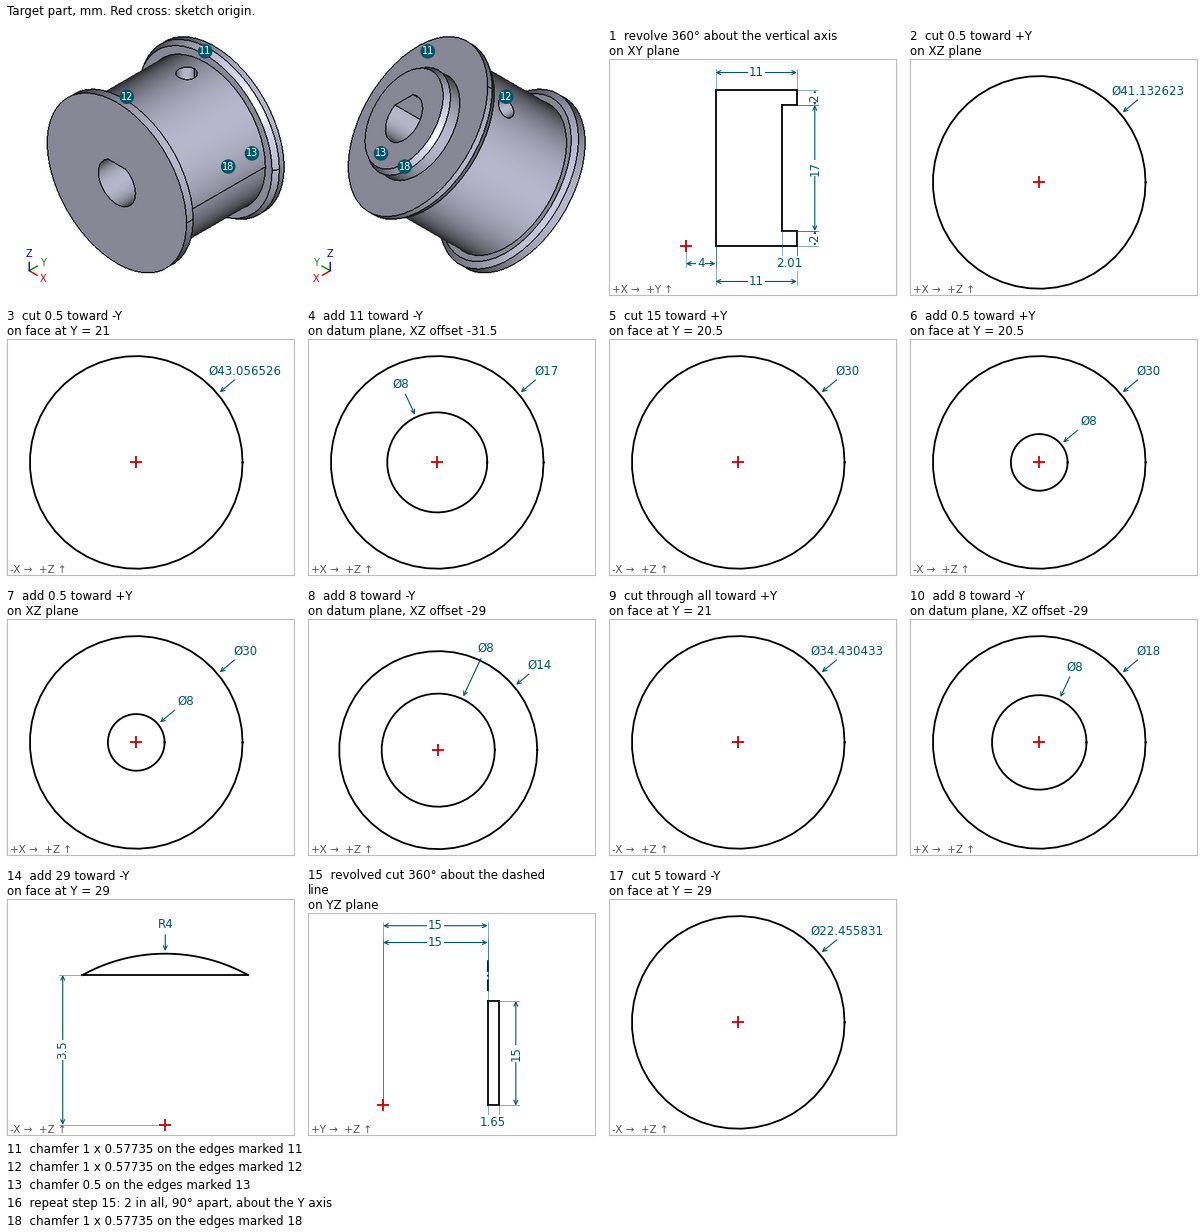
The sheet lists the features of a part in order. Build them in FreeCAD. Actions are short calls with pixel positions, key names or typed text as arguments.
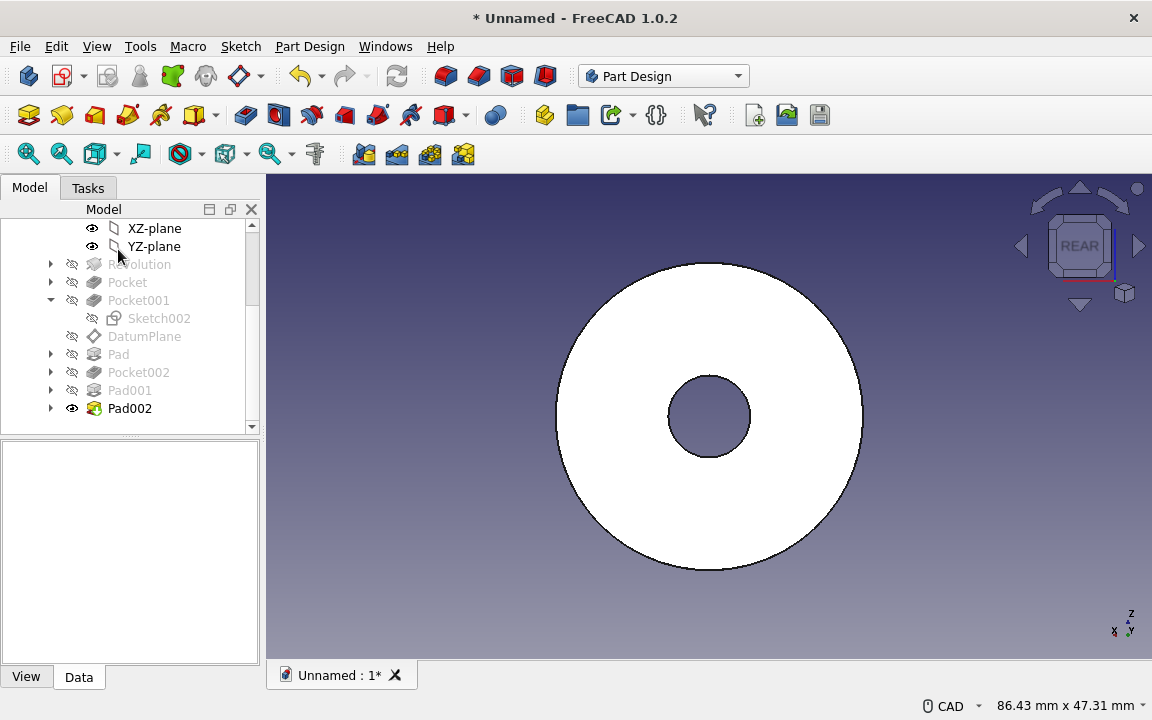
scroll(161, 314, down, 3)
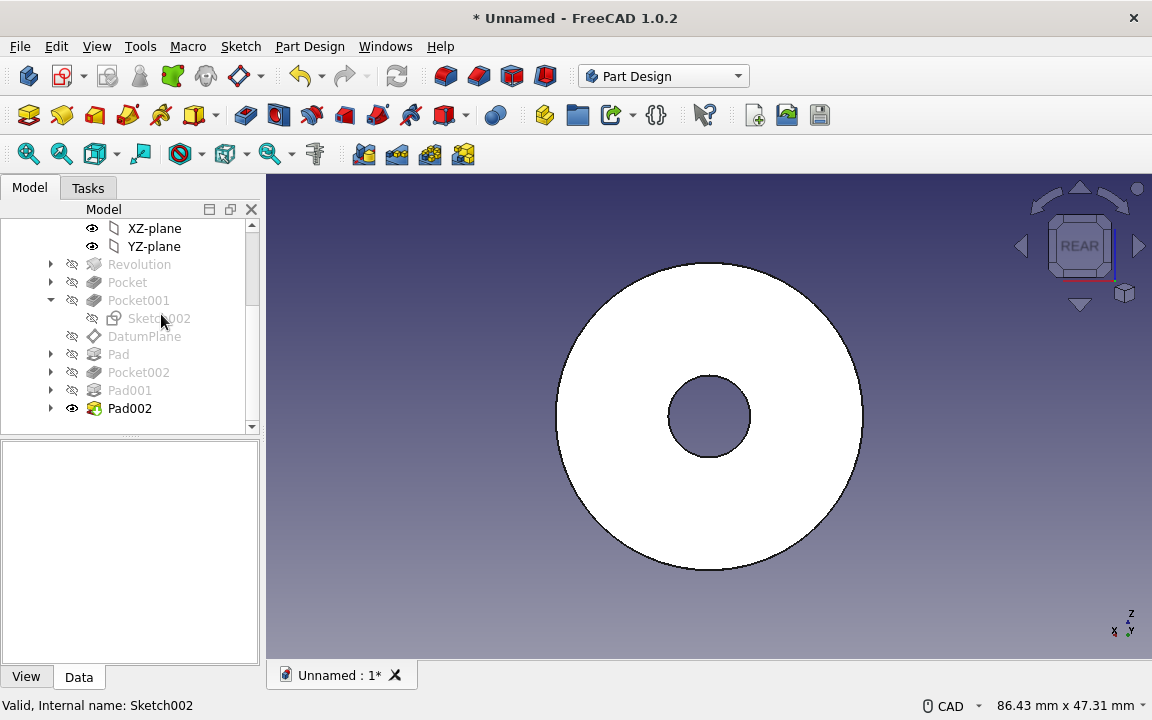
scroll(161, 314, up, 15)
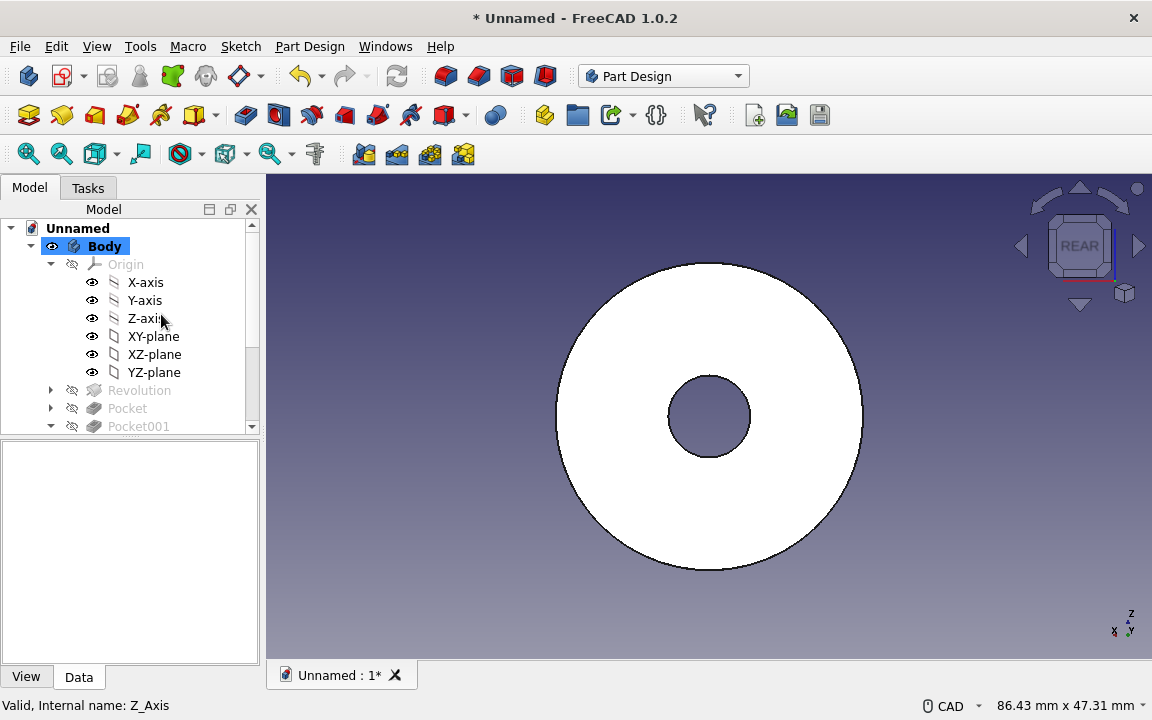
click(137, 354)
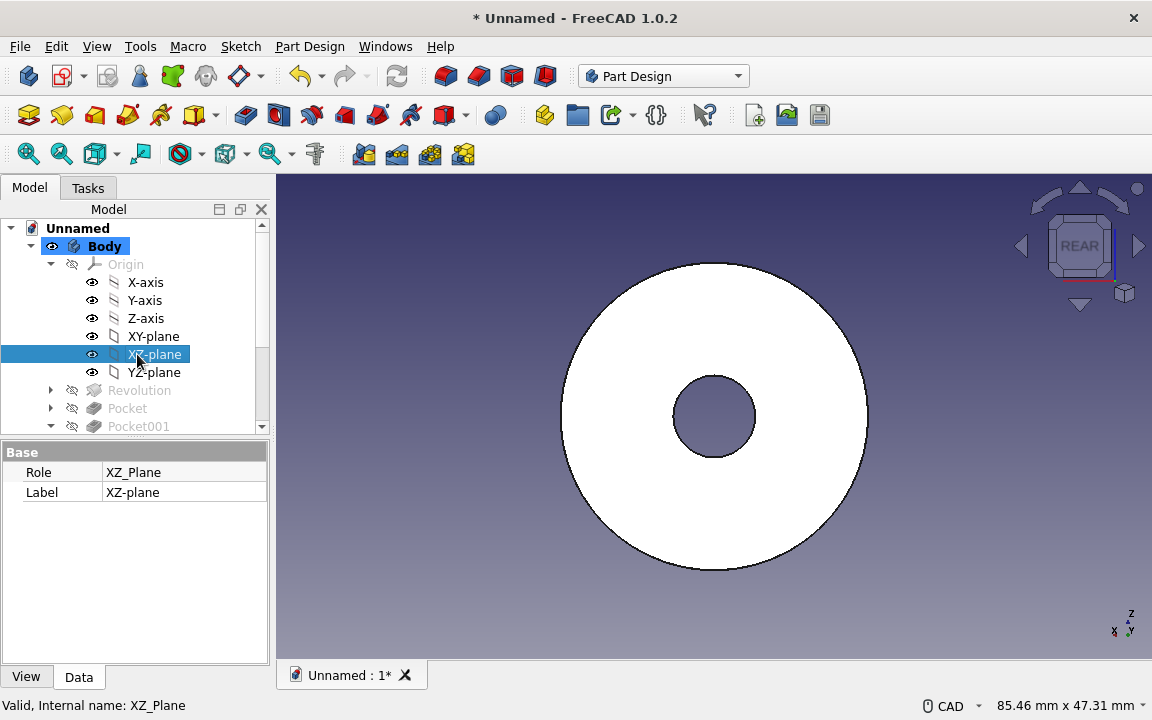
click(238, 76)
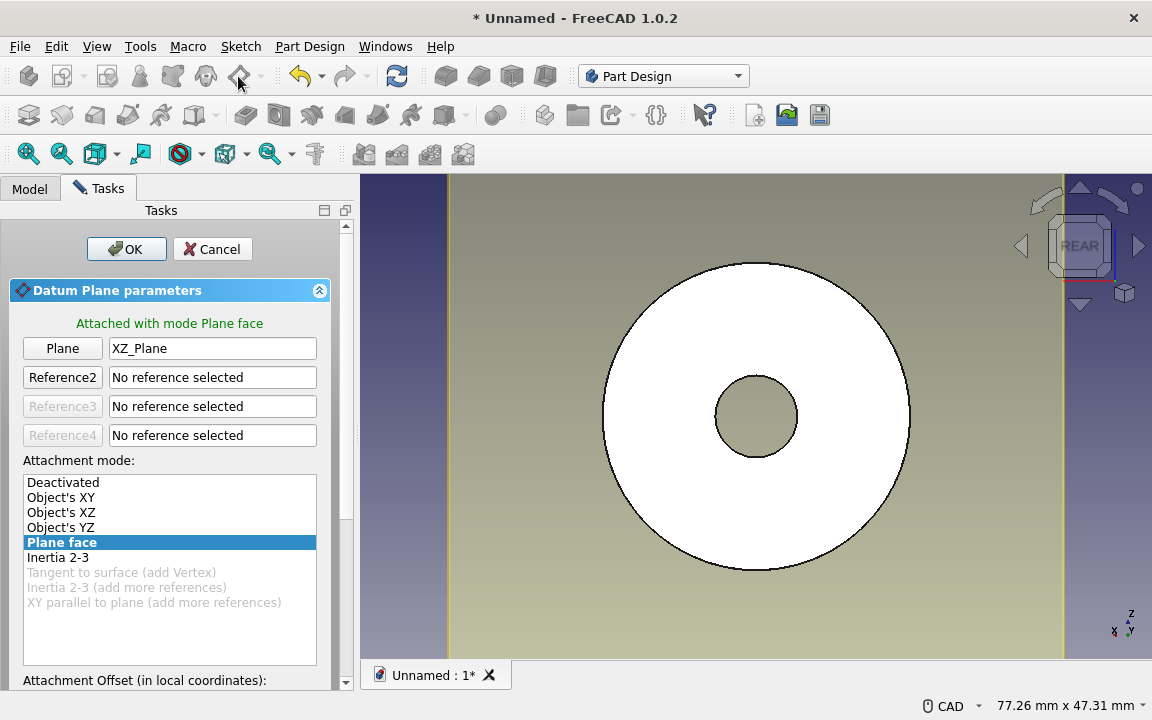
scroll(346, 455, down, 3)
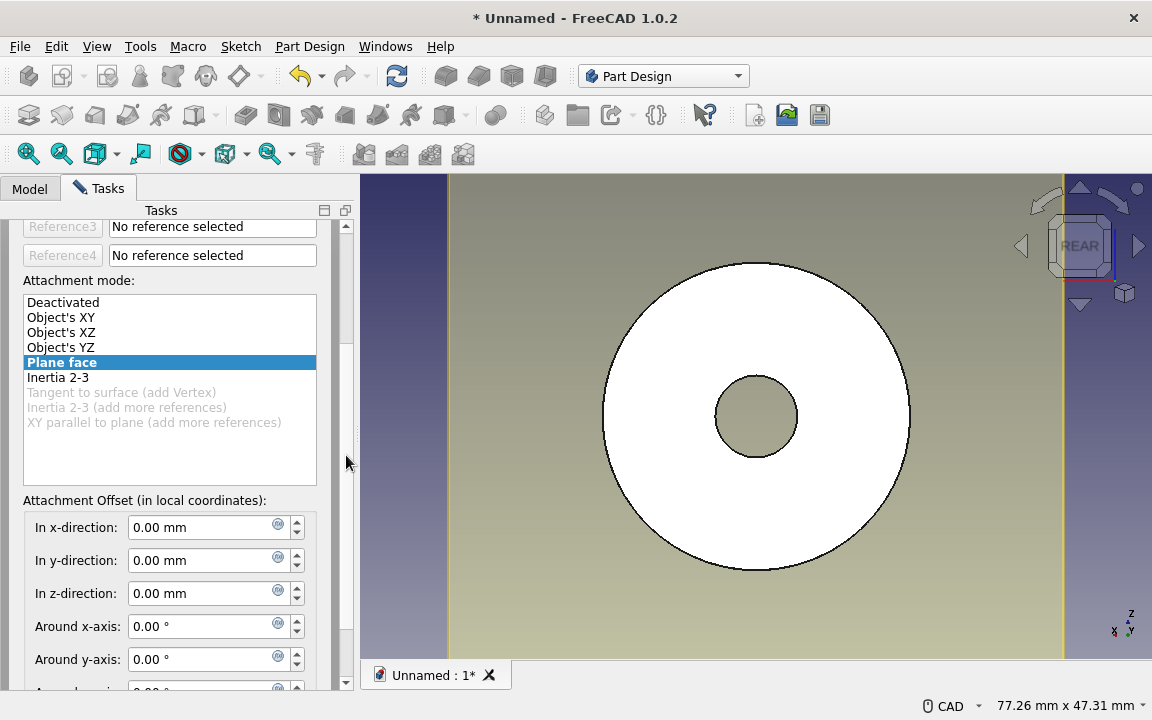
triple_click(210, 594)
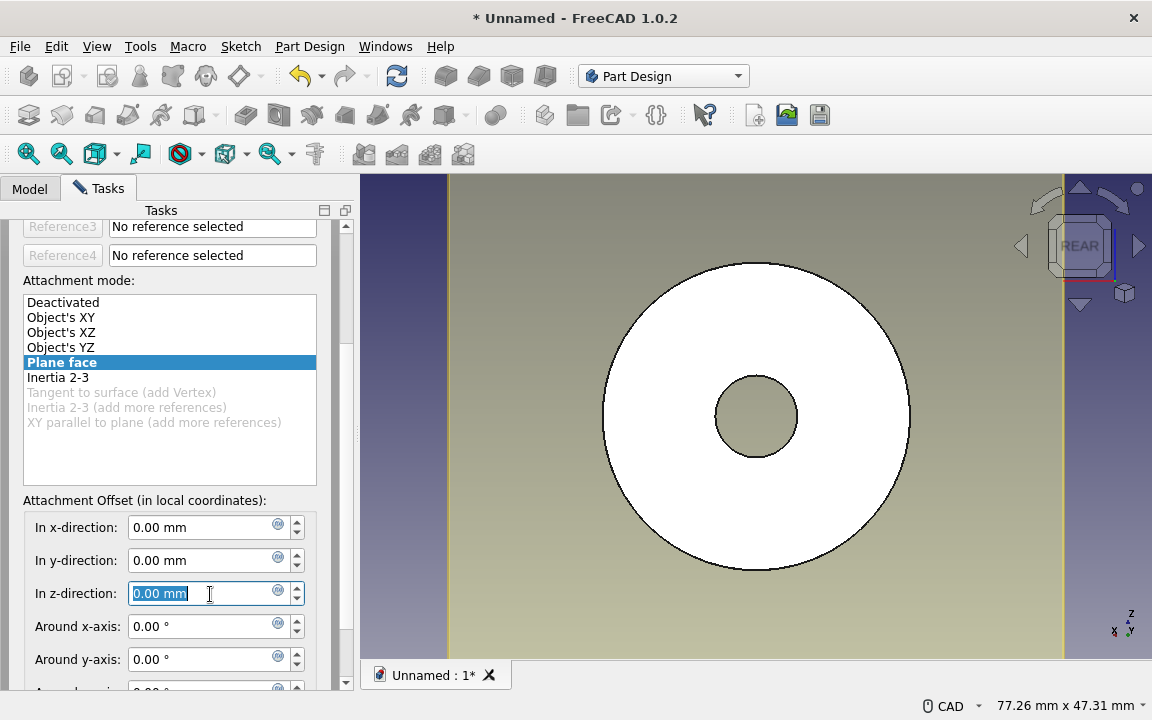
text(-29)
key(Tab)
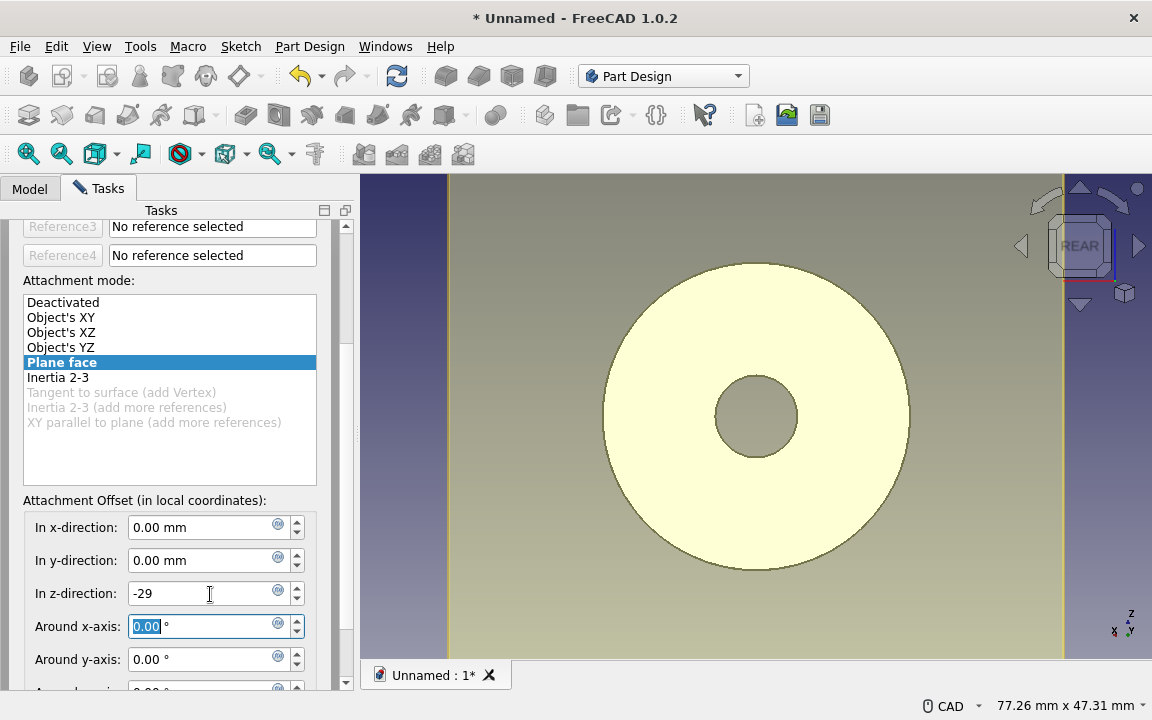
scroll(346, 455, up, 4)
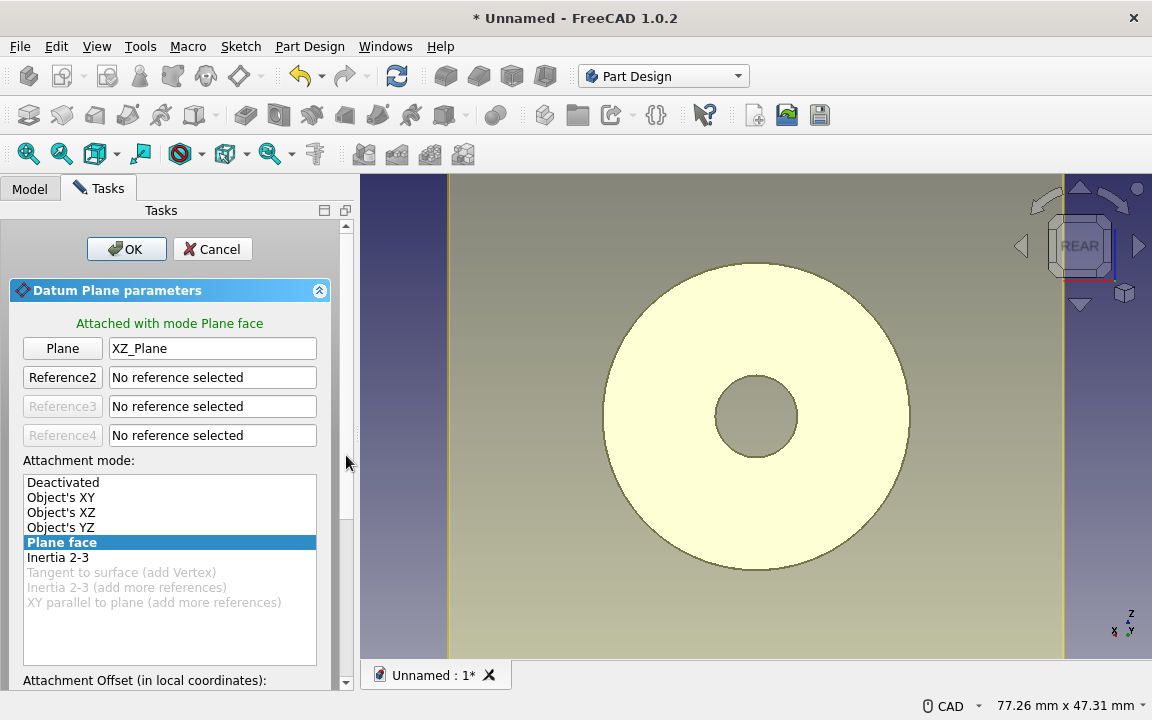
click(127, 249)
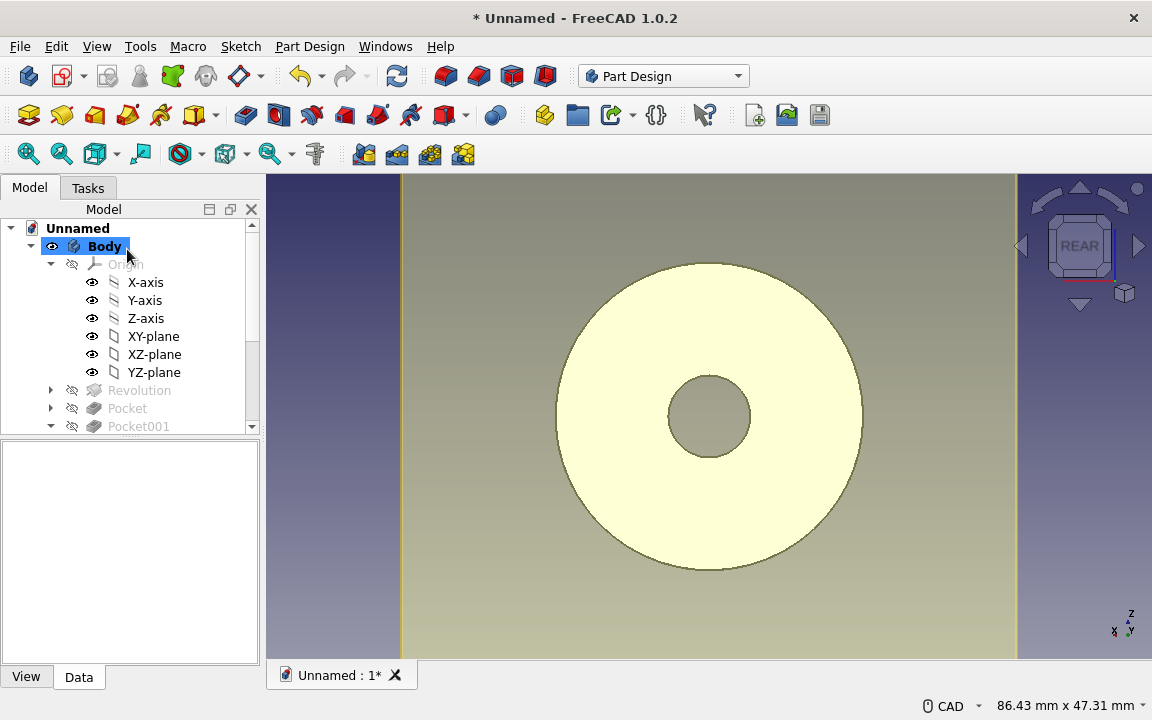
scroll(101, 332, down, 3)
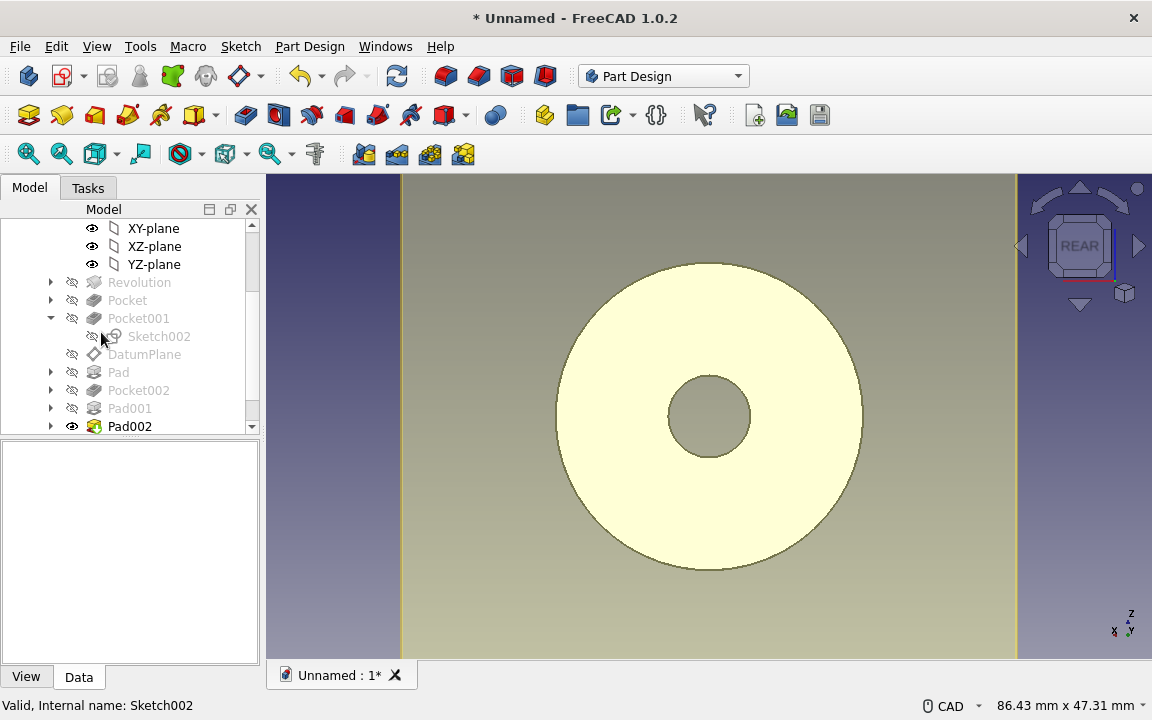
click(117, 408)